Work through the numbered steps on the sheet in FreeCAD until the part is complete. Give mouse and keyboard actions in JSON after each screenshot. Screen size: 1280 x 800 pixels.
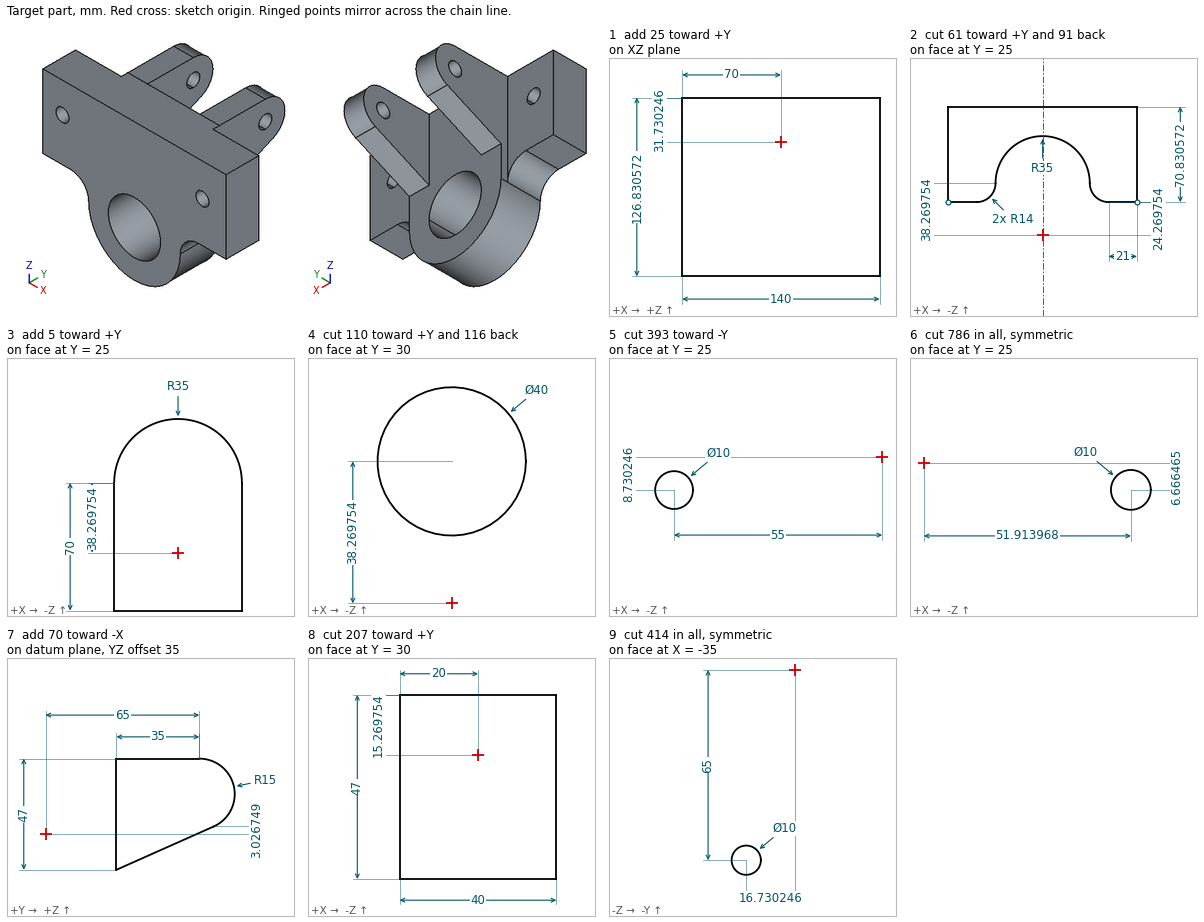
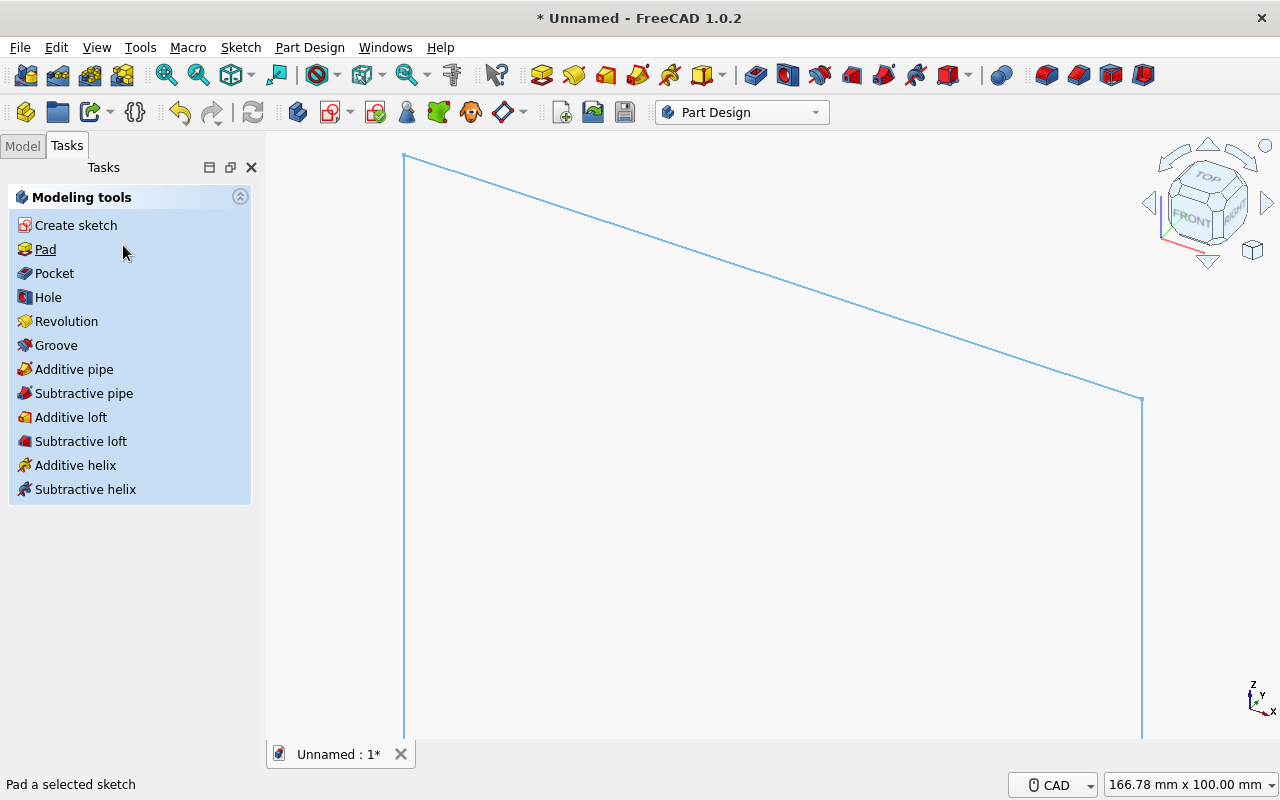
{"action": "left_click", "coordinate": [542, 76]}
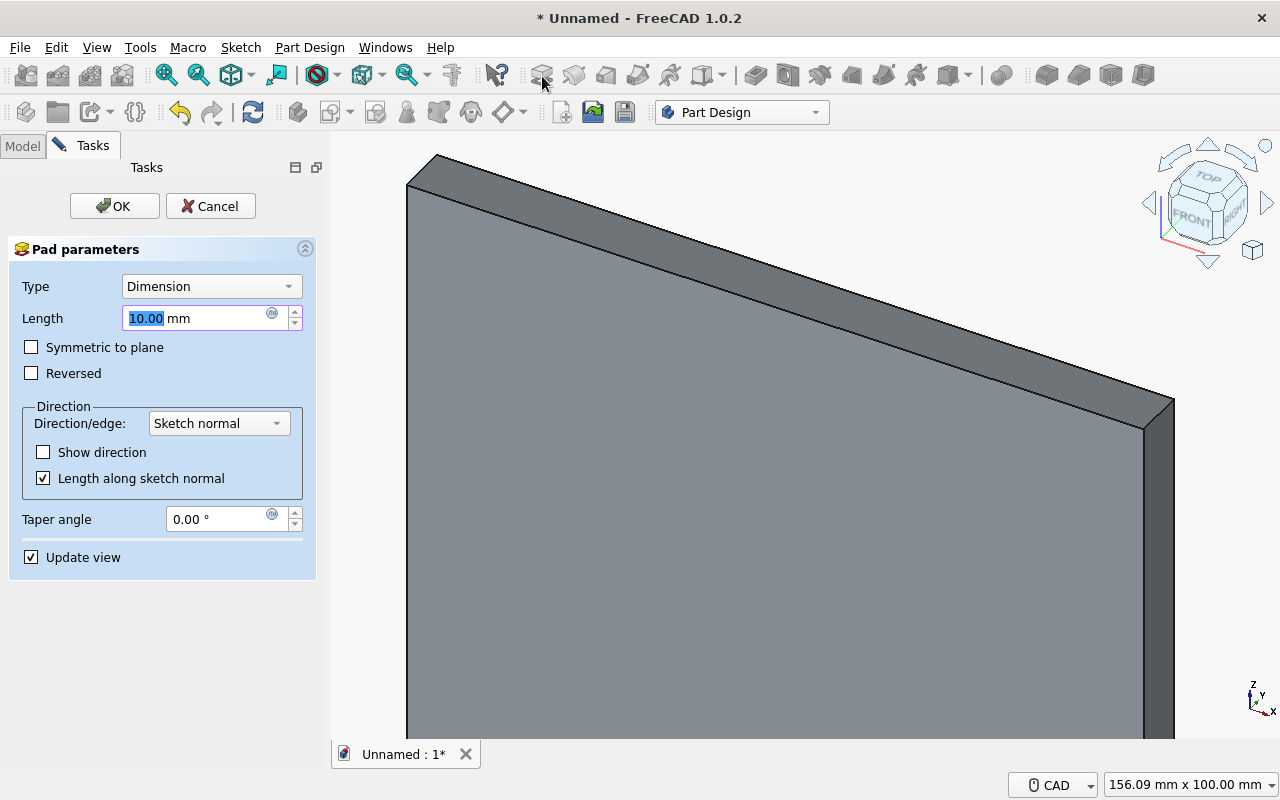
{"action": "type", "text": "25"}
{"action": "key", "text": "Tab"}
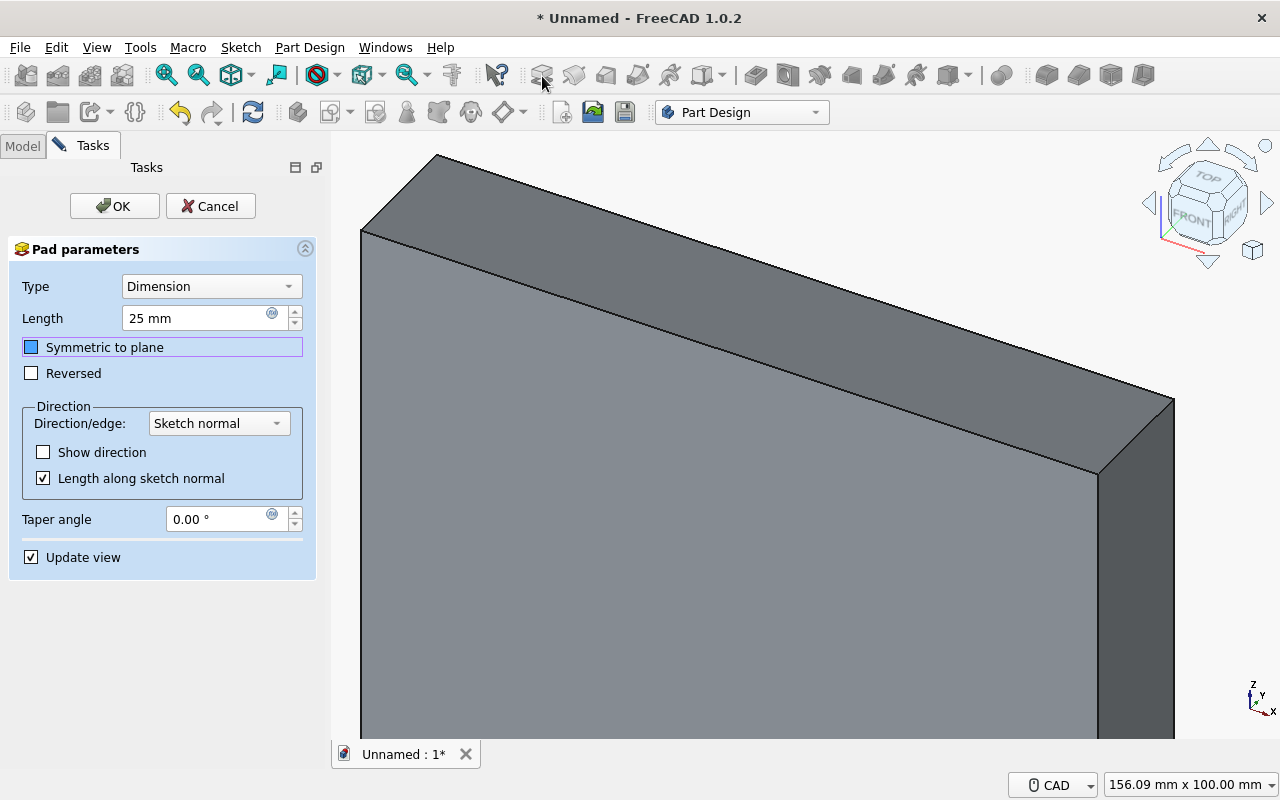
{"action": "left_click", "coordinate": [30, 373]}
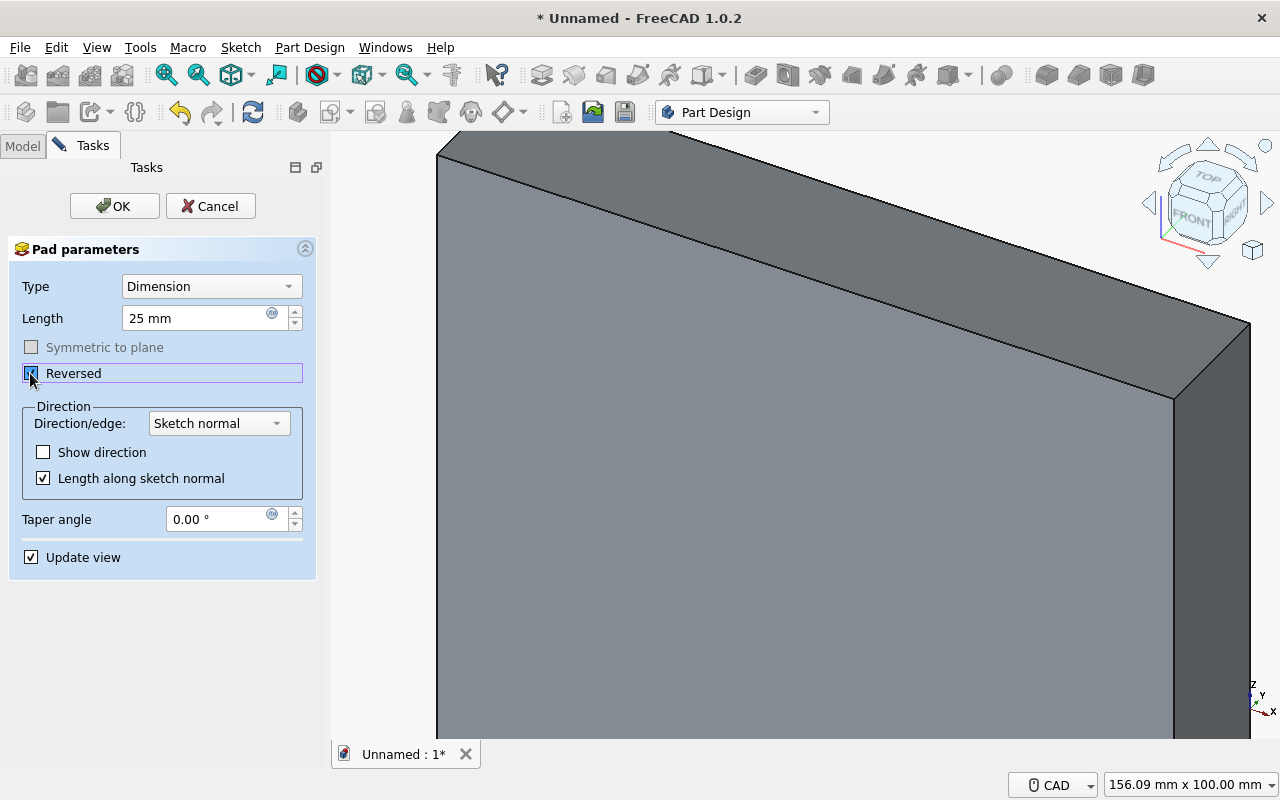
{"action": "left_click", "coordinate": [115, 206]}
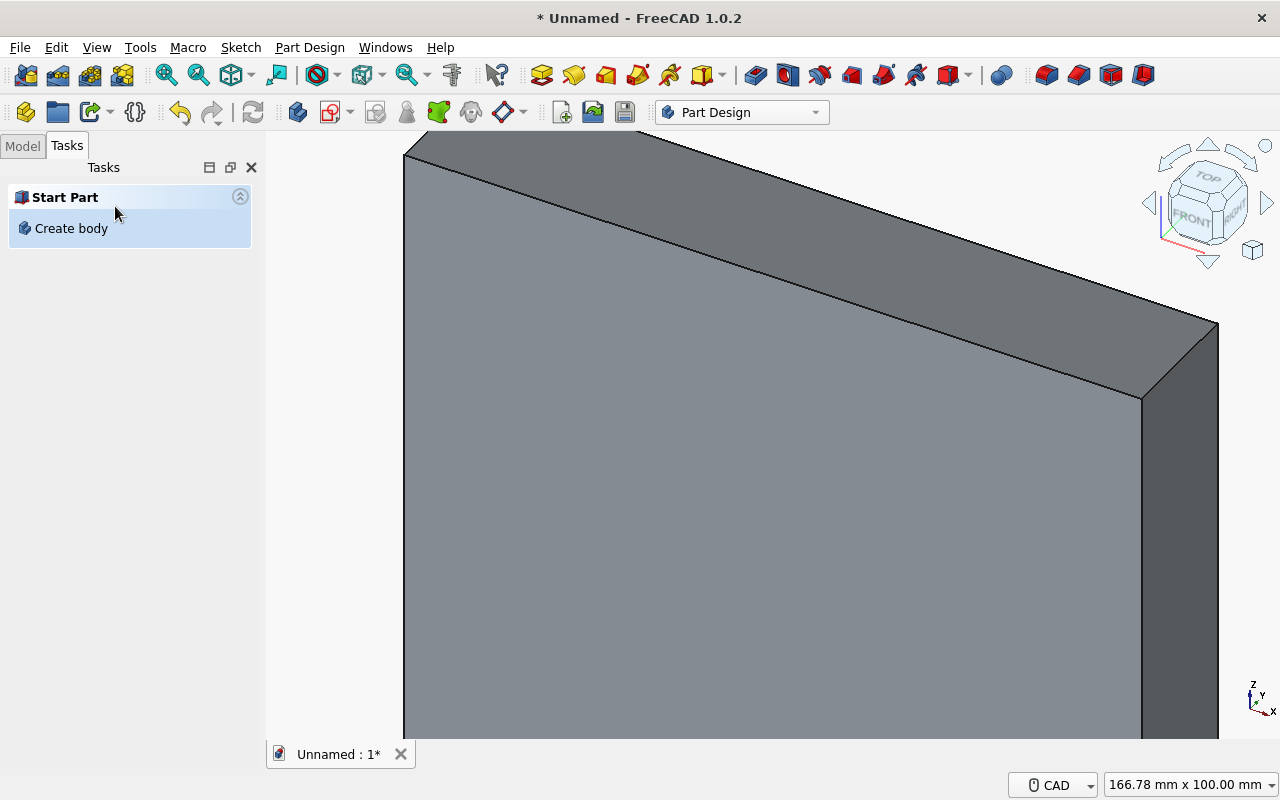
{"action": "left_click", "coordinate": [168, 76]}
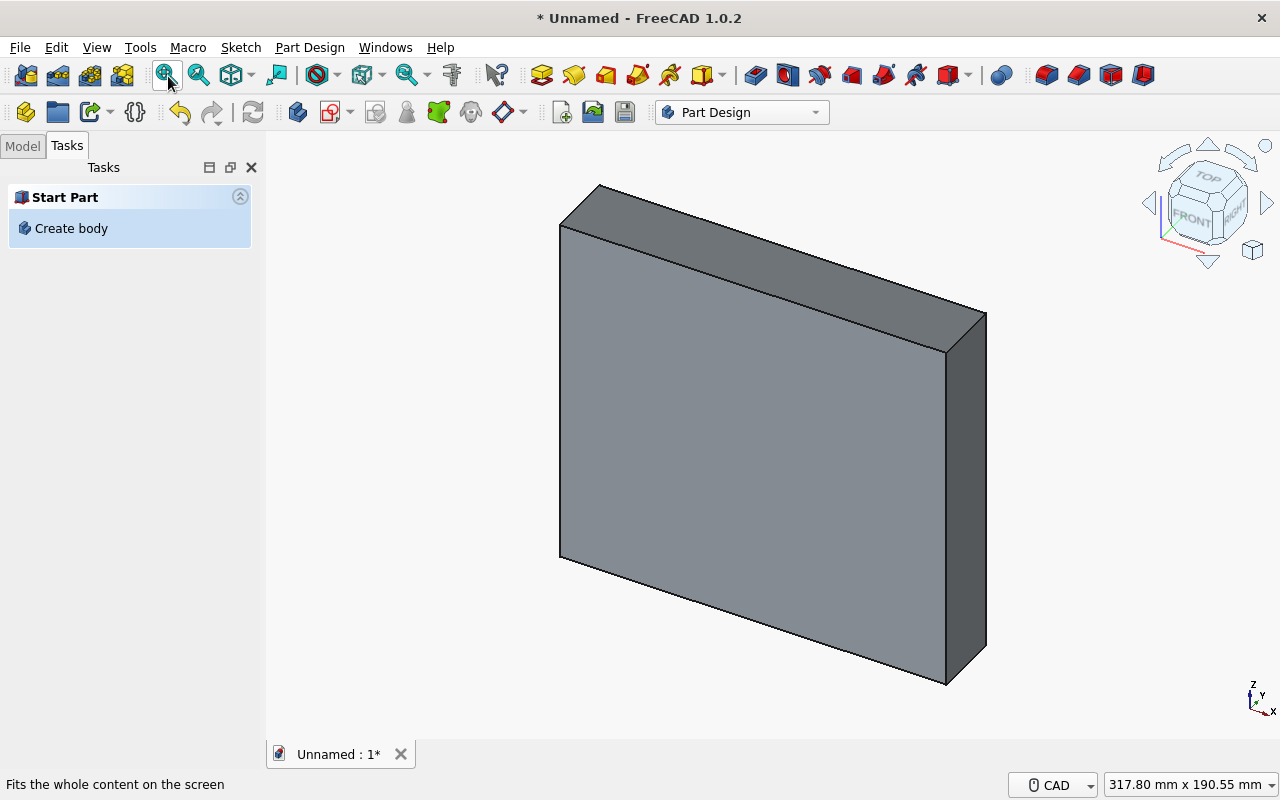
{"action": "key", "text": "4"}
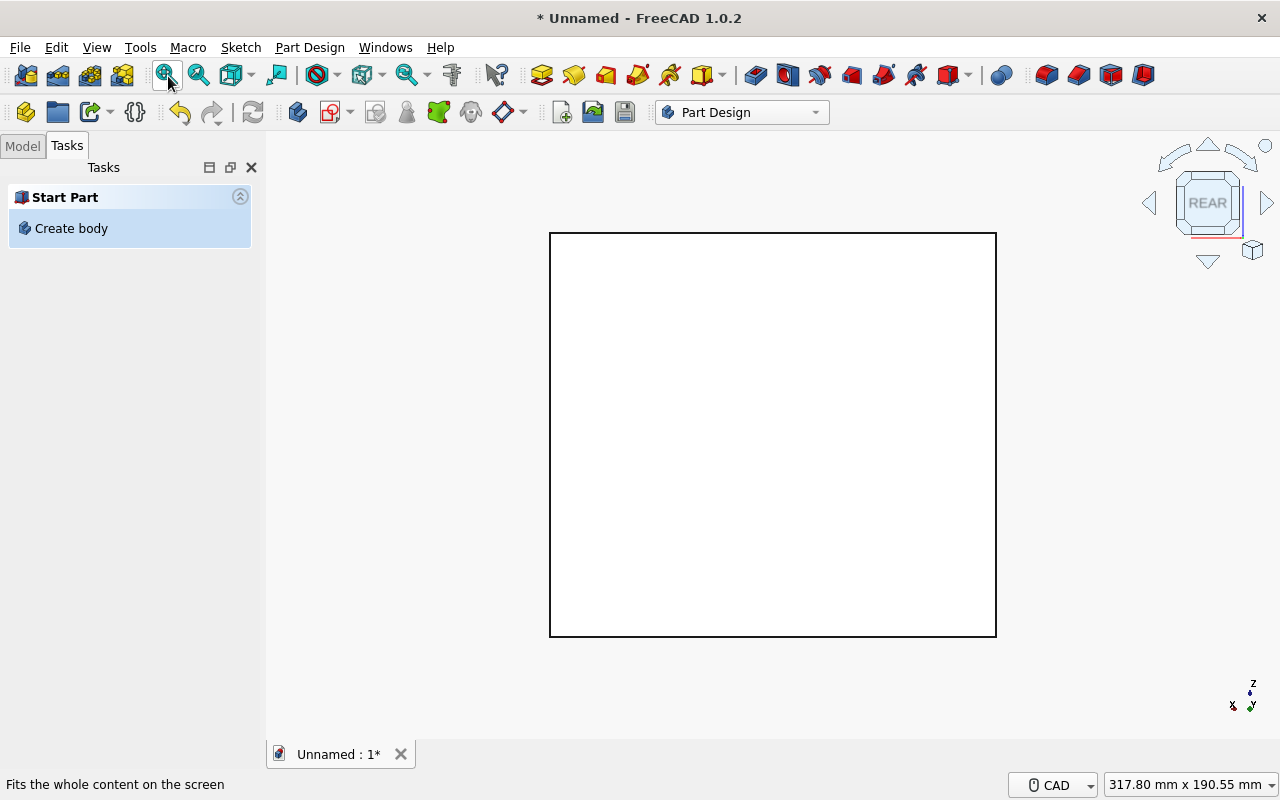
{"action": "left_click", "coordinate": [773, 434]}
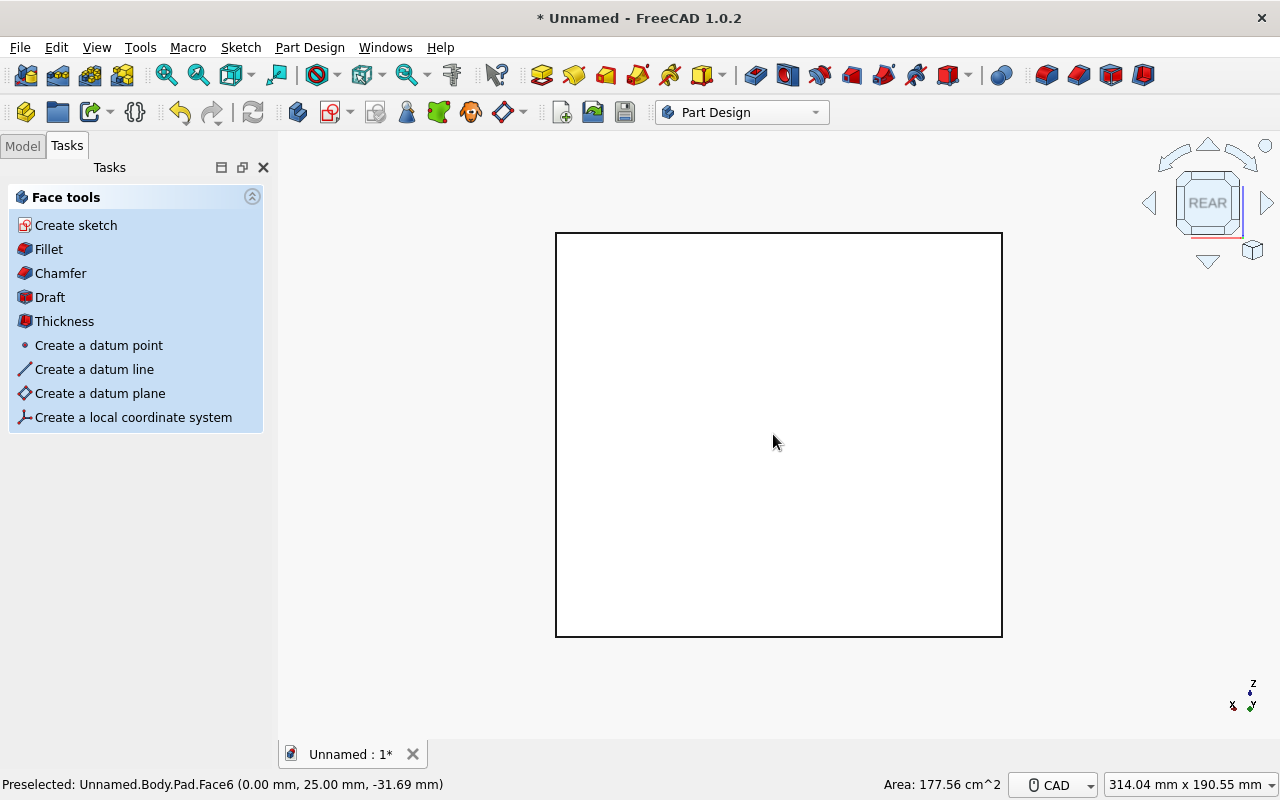
{"action": "left_click", "coordinate": [330, 112]}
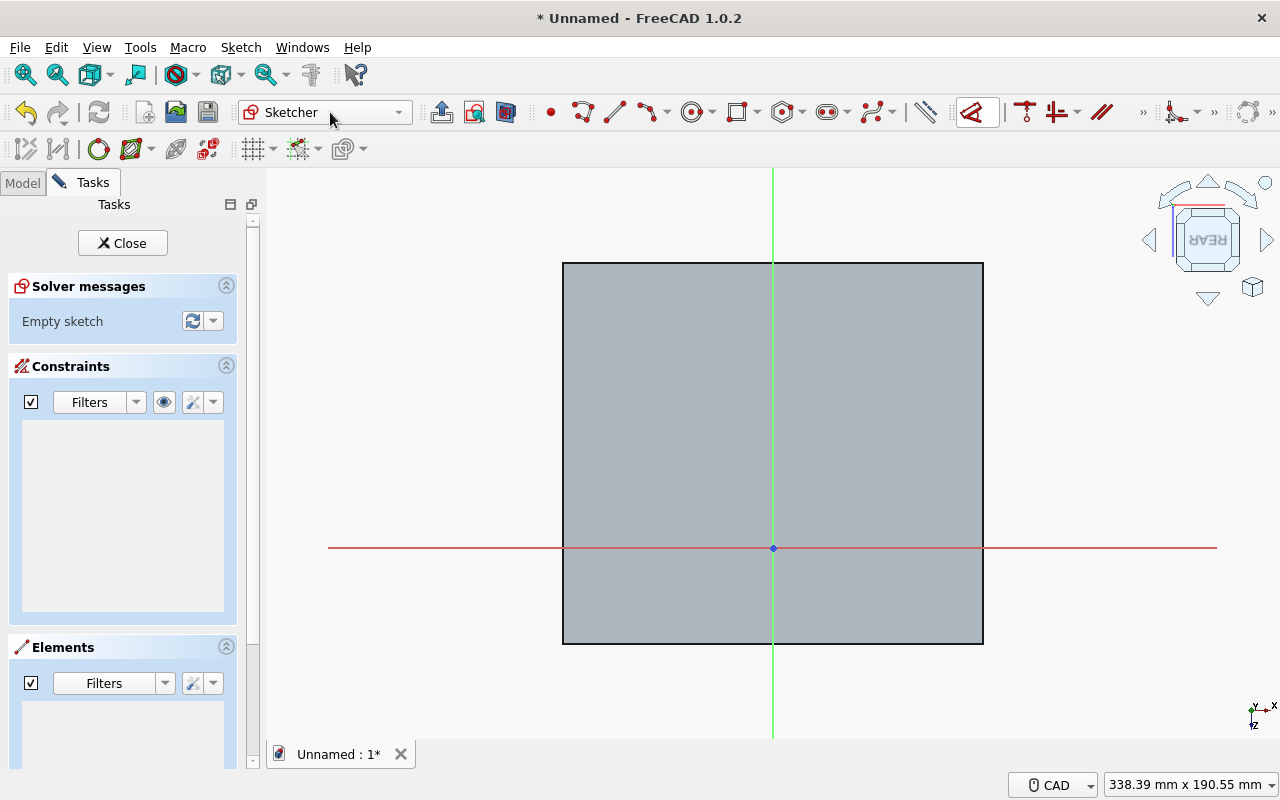
{"action": "left_click", "coordinate": [584, 112]}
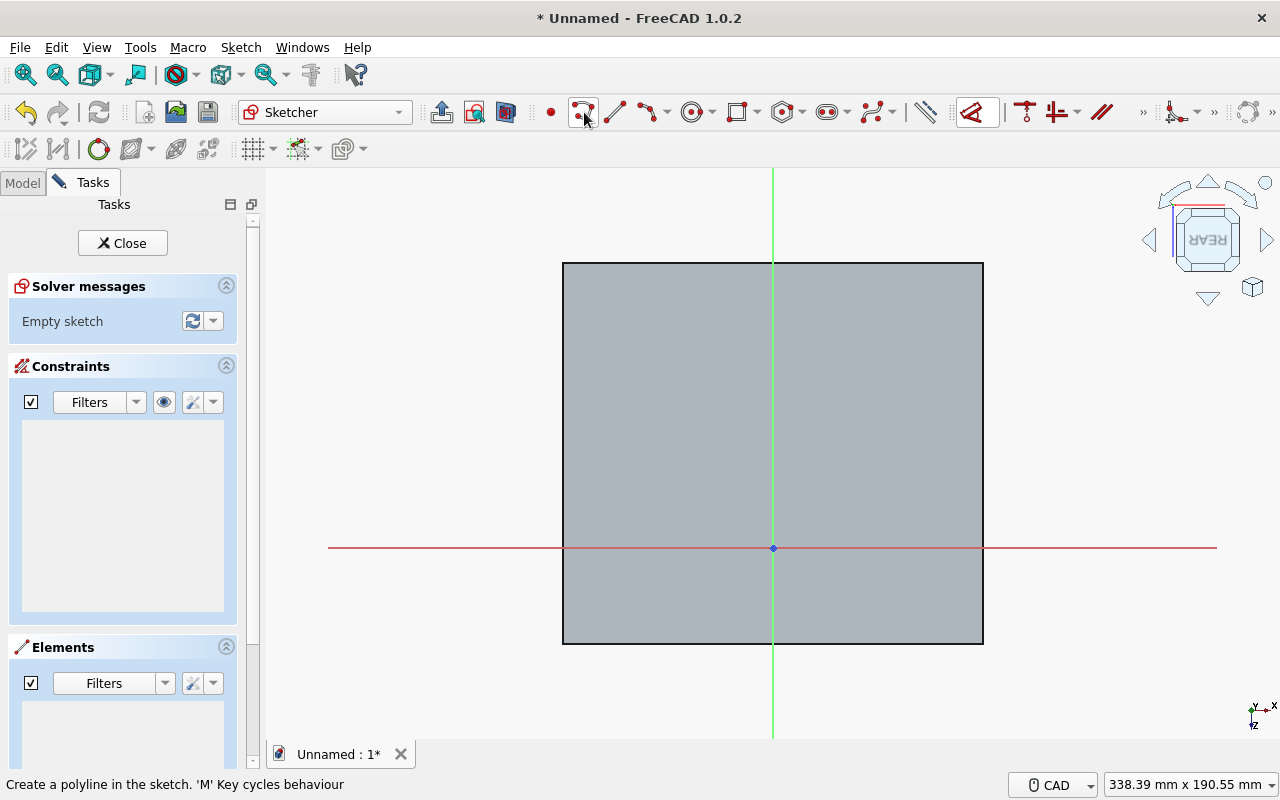
{"action": "left_click", "coordinate": [920, 476]}
{"action": "left_click", "coordinate": [983, 476]}
{"action": "left_click", "coordinate": [983, 263]}
{"action": "left_click", "coordinate": [563, 263]}
{"action": "left_click", "coordinate": [563, 476]}
{"action": "left_click", "coordinate": [626, 476]}
{"action": "right_click", "coordinate": [626, 476]}